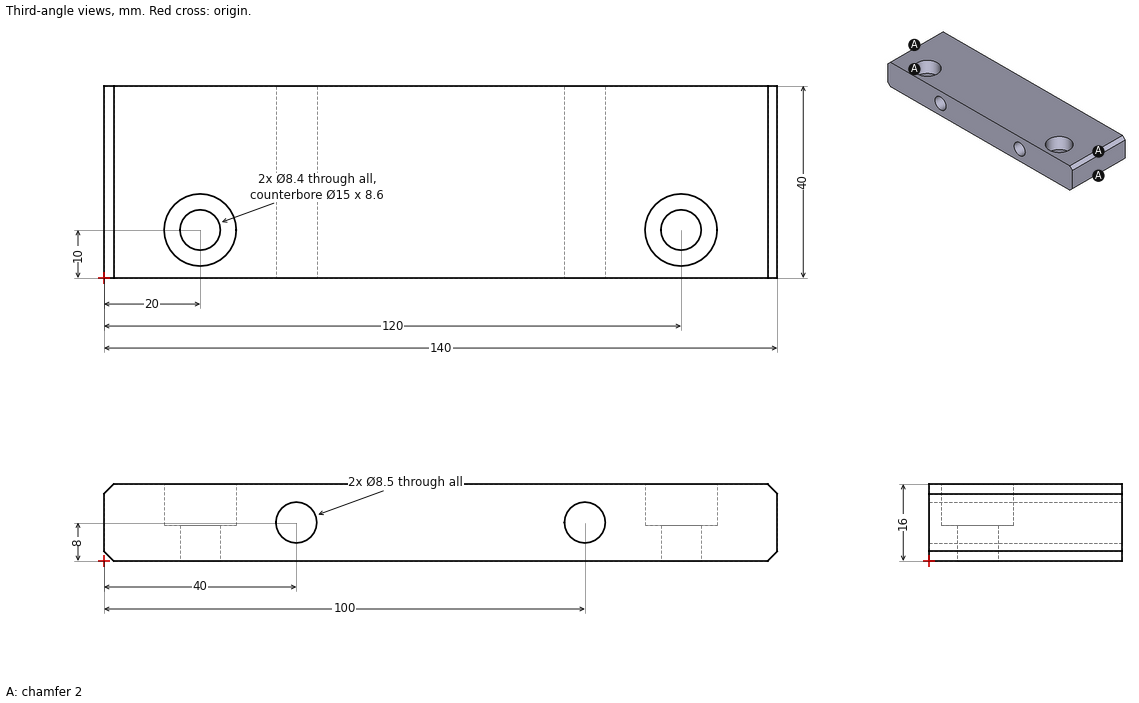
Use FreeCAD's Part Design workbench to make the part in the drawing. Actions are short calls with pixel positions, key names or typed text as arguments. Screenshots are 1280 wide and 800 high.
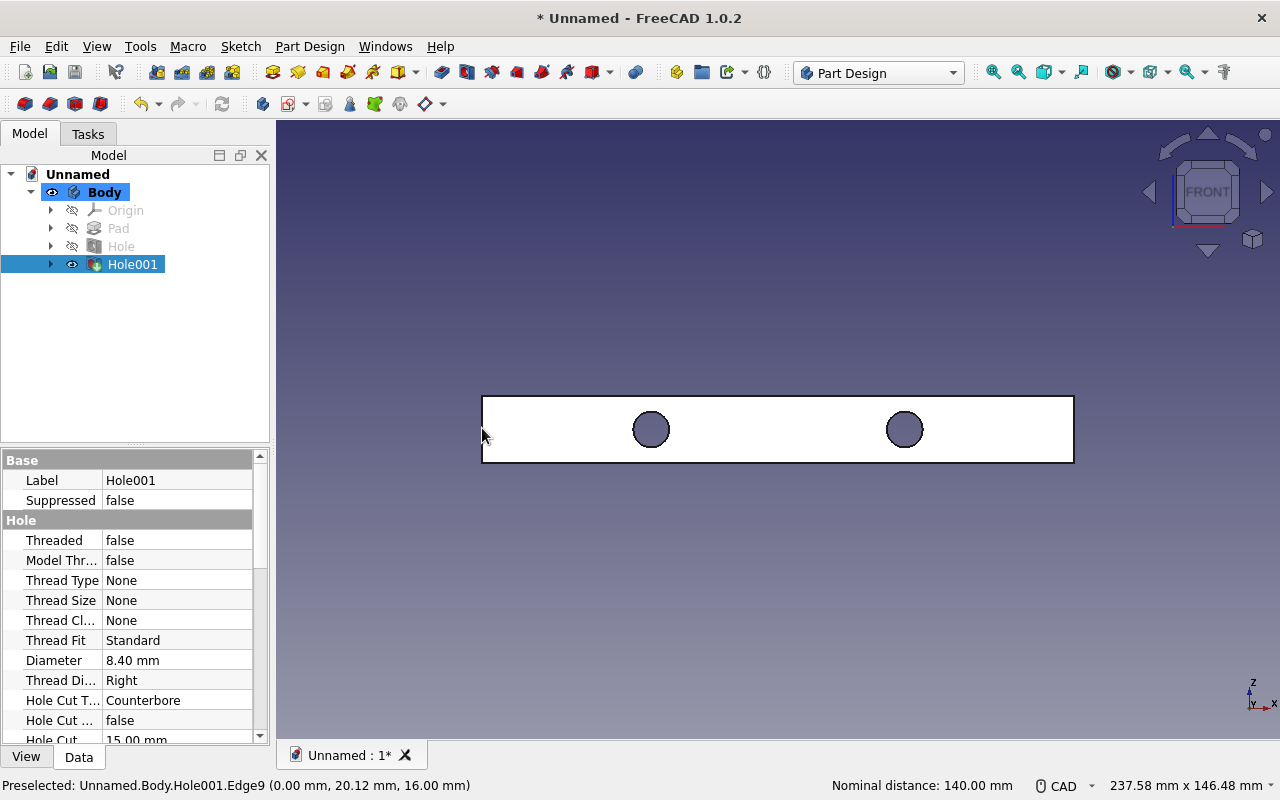
key(3)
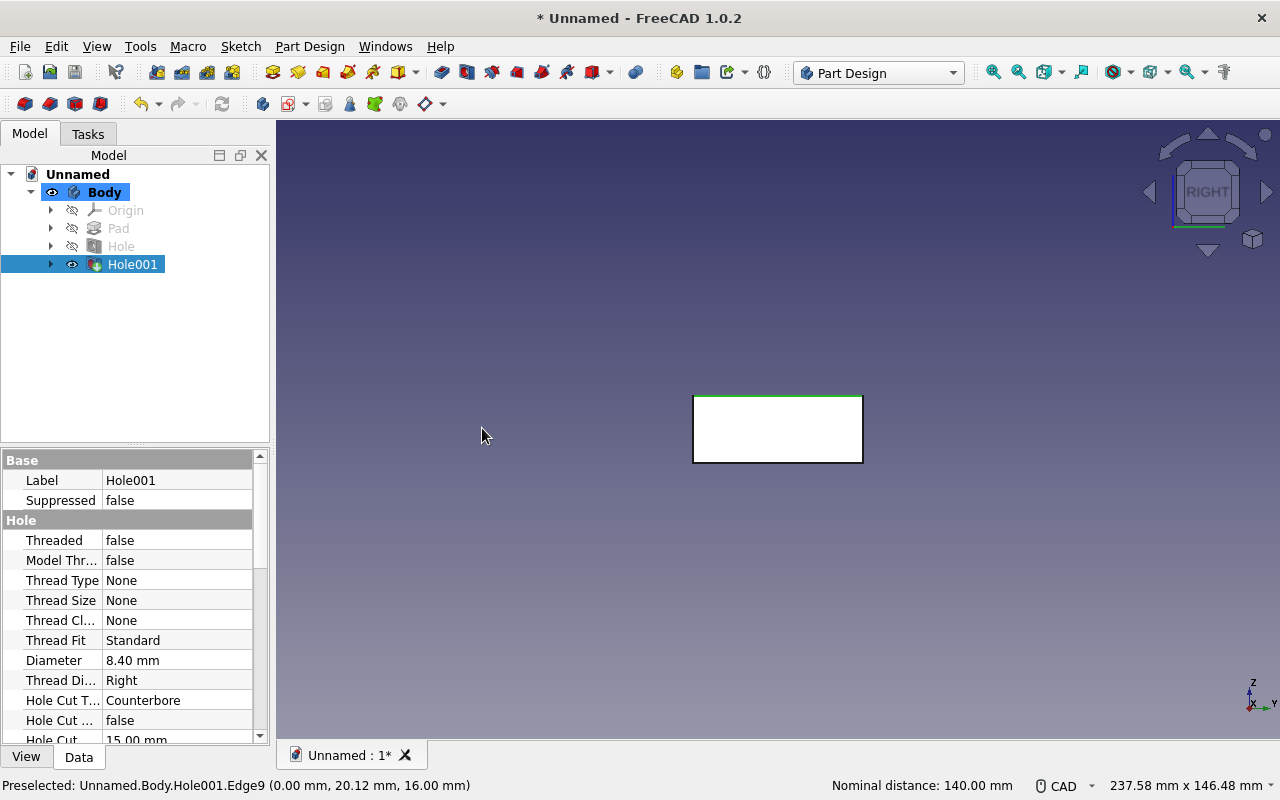
click(994, 72)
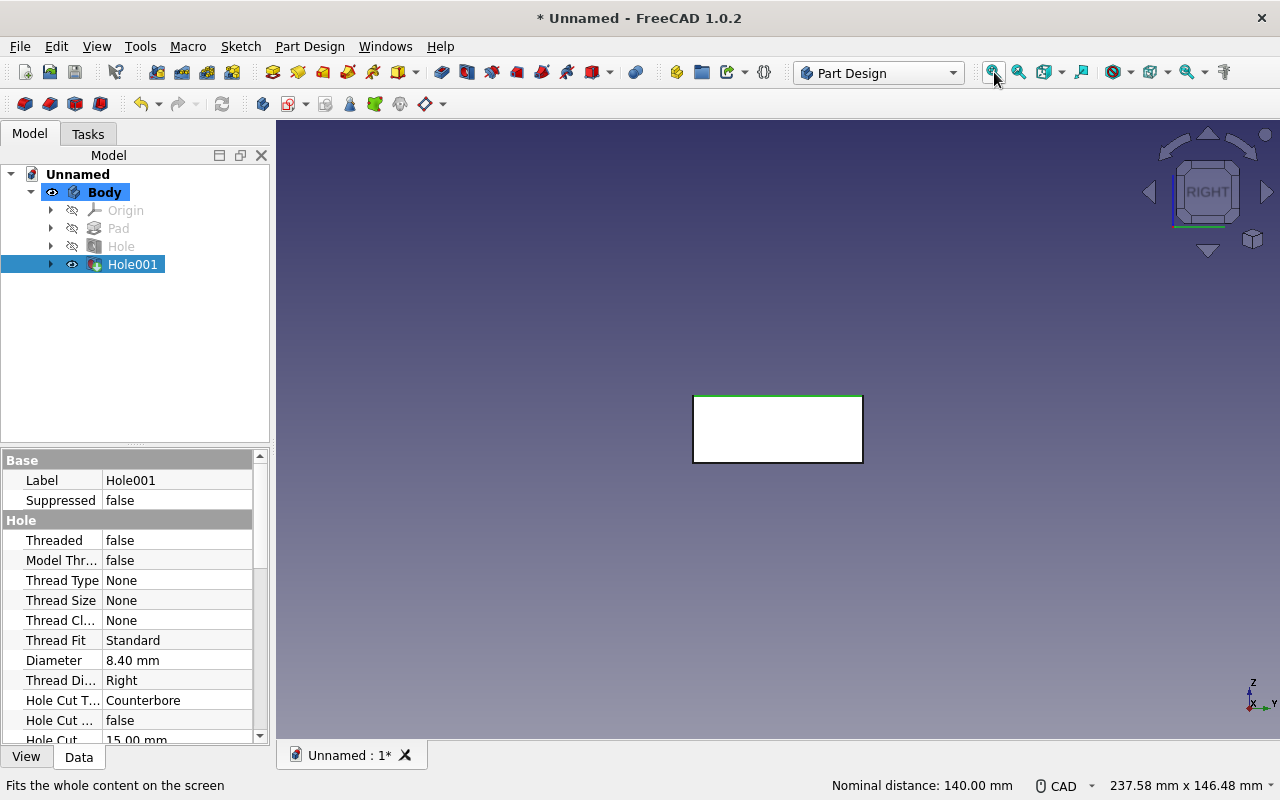
click(778, 462, ctrl)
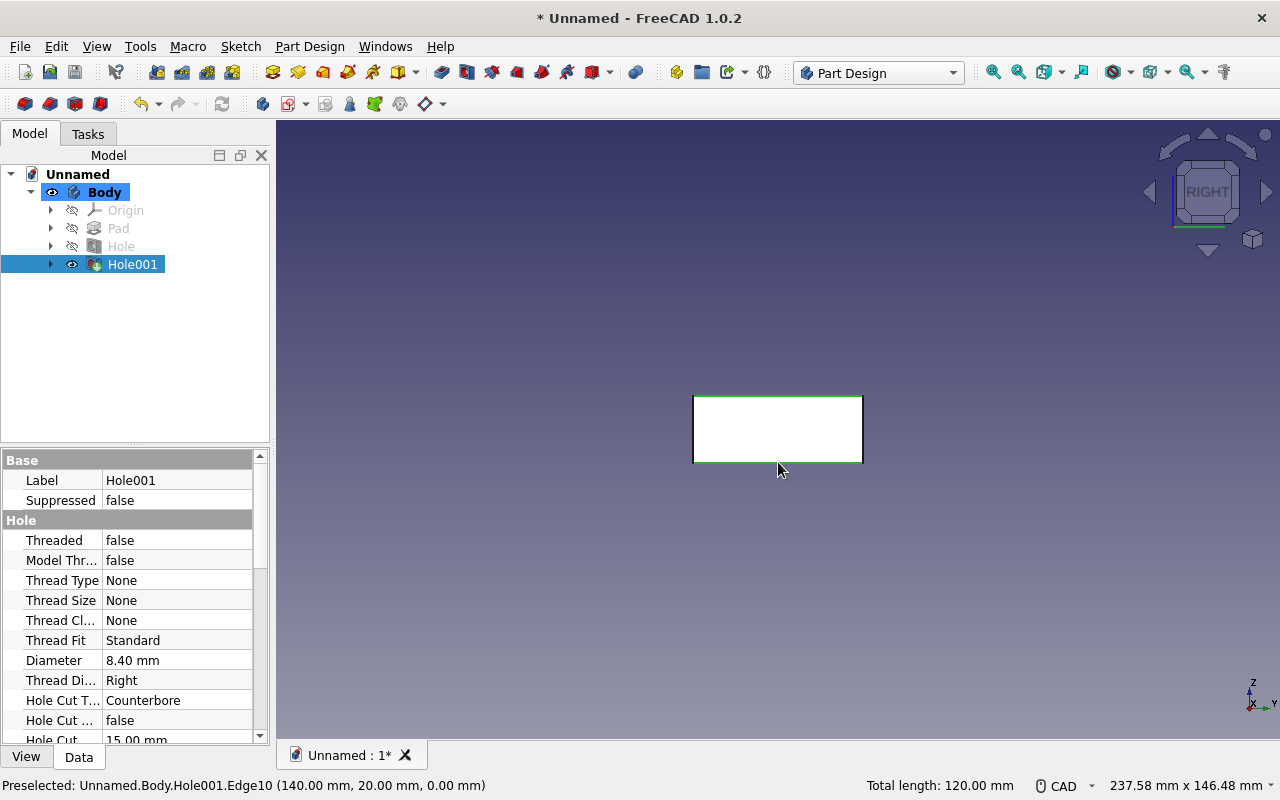
key(5)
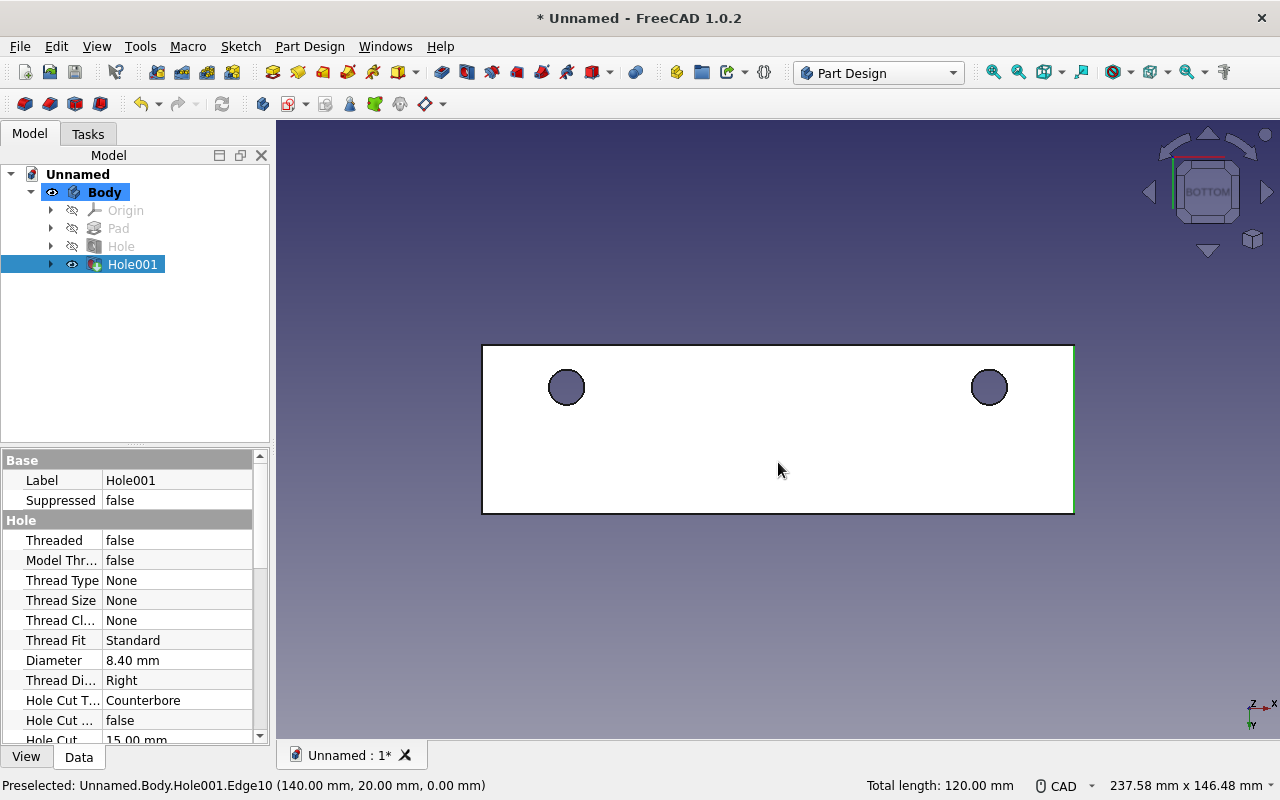
click(482, 428, ctrl)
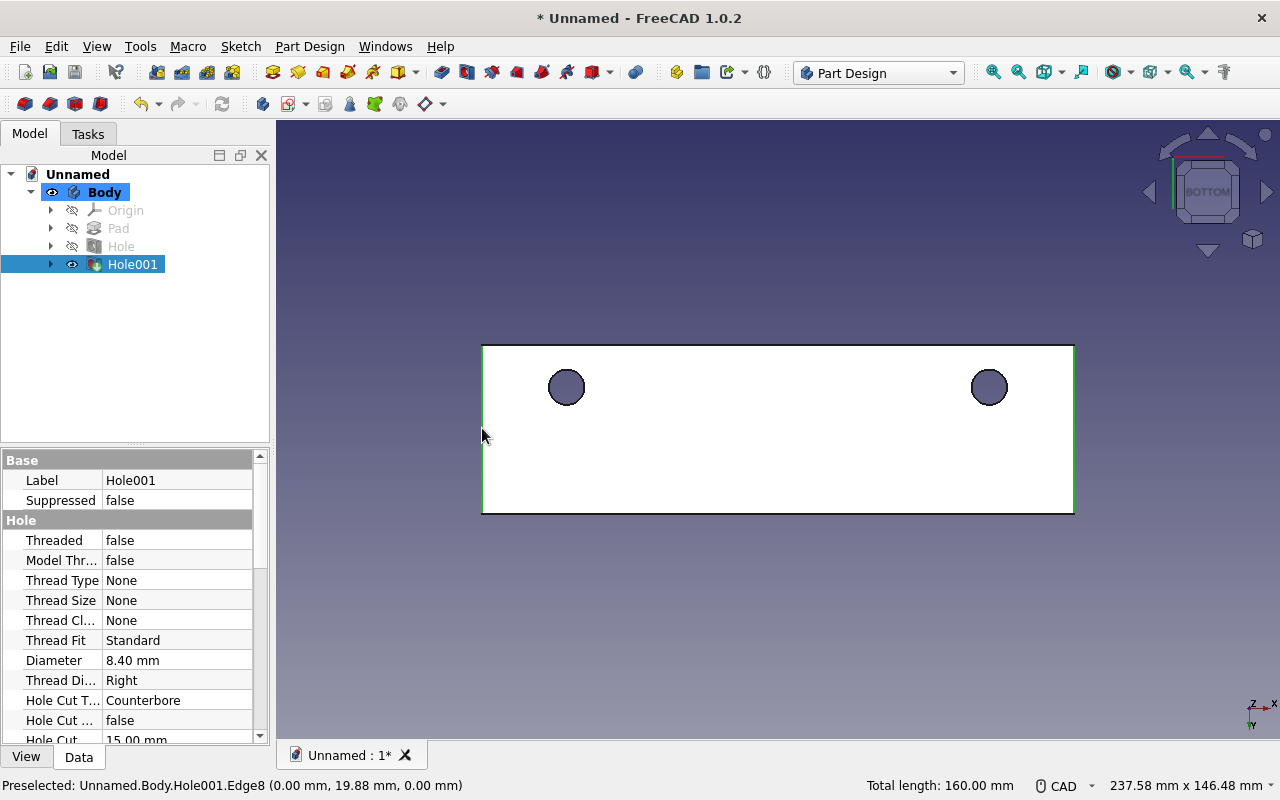
click(50, 104)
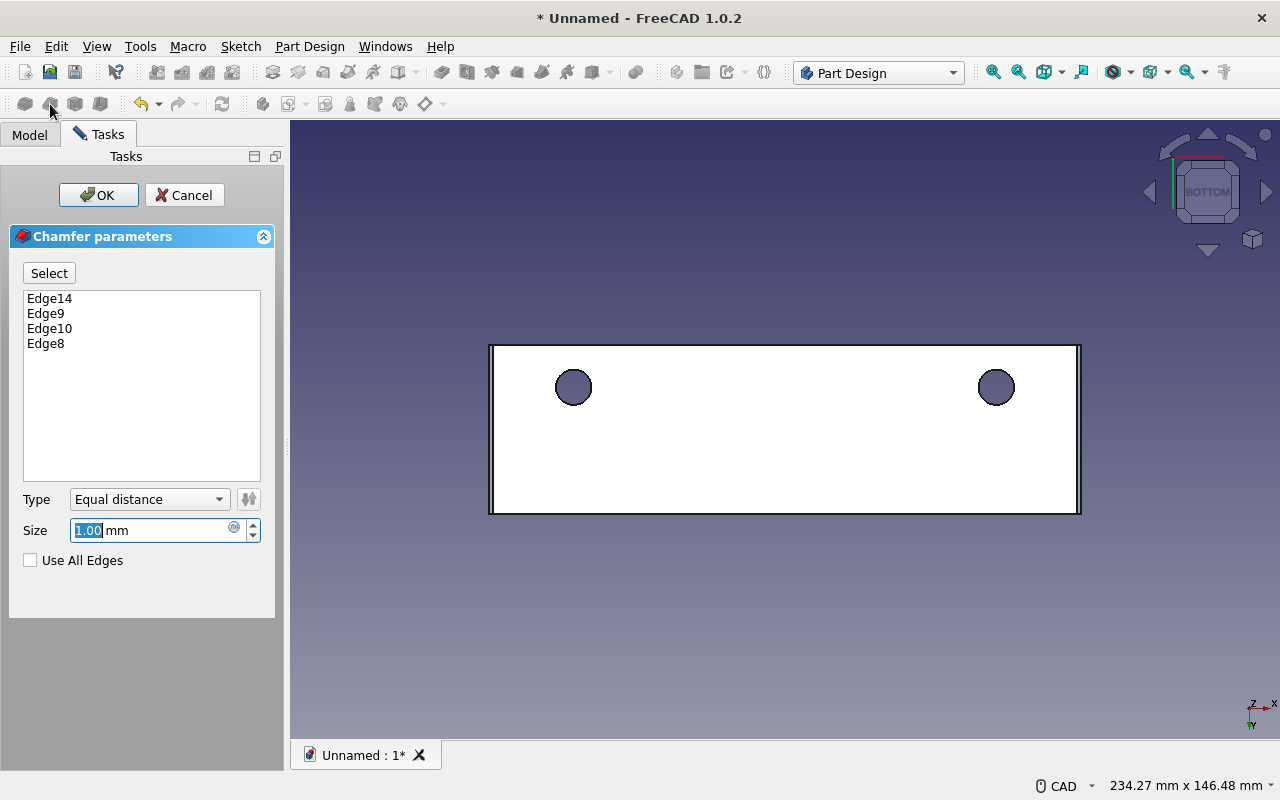
text(2)
key(Tab)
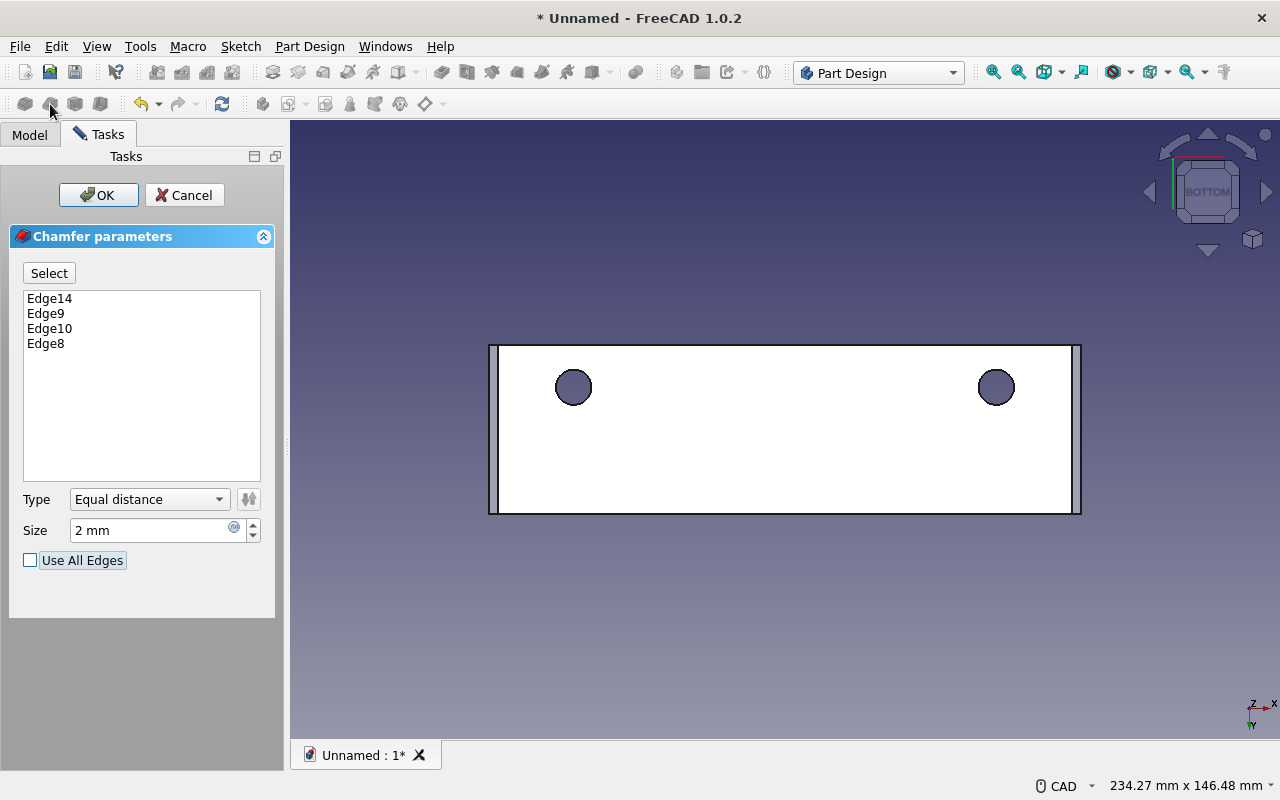
click(99, 195)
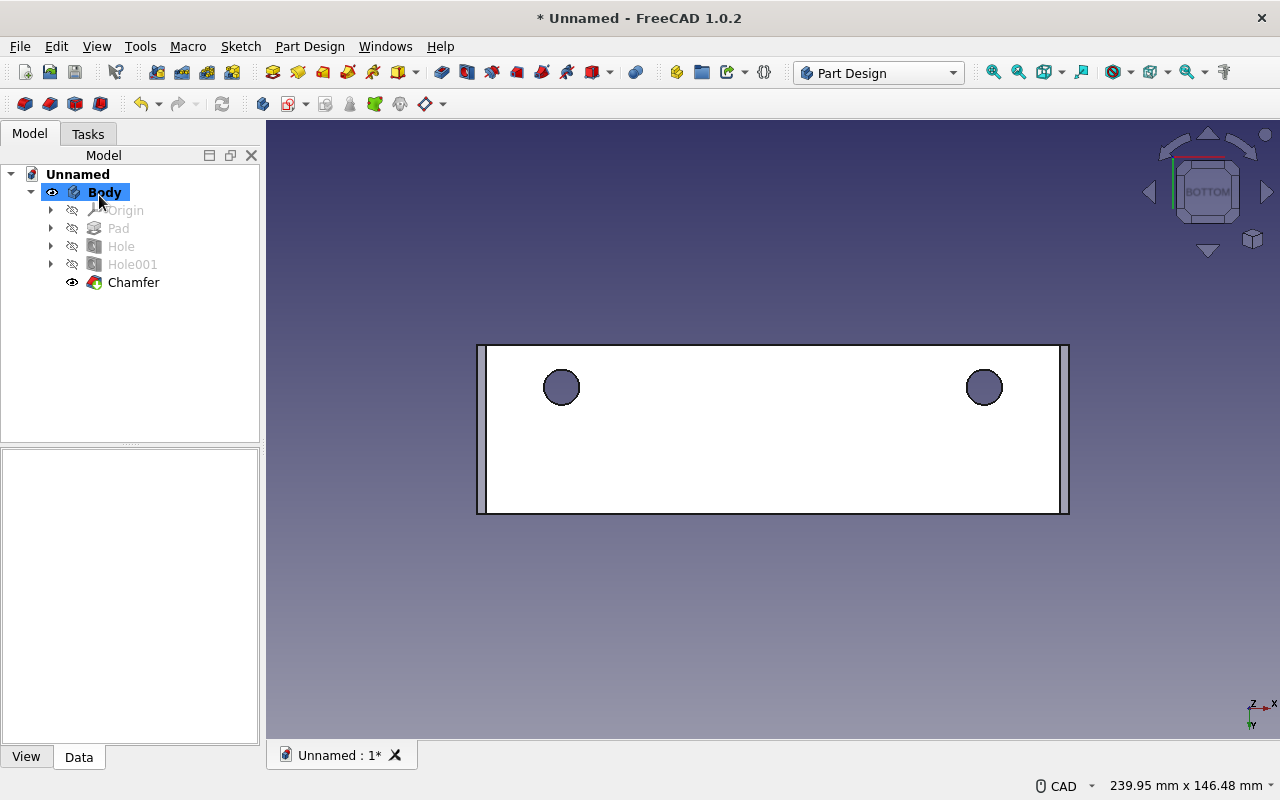
key(0)